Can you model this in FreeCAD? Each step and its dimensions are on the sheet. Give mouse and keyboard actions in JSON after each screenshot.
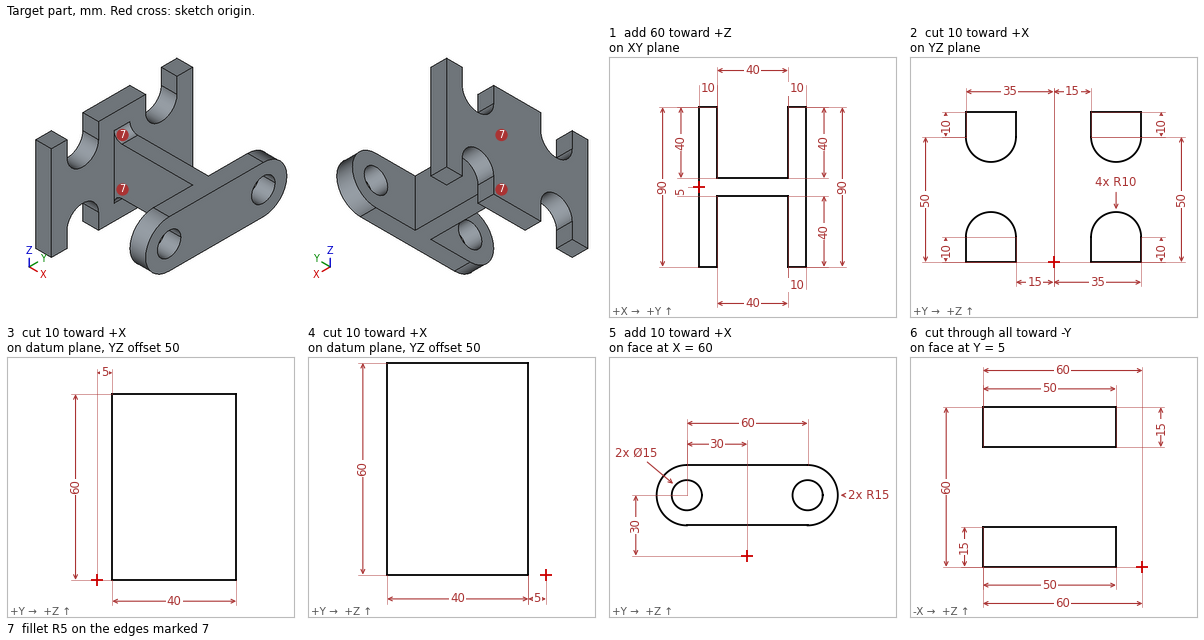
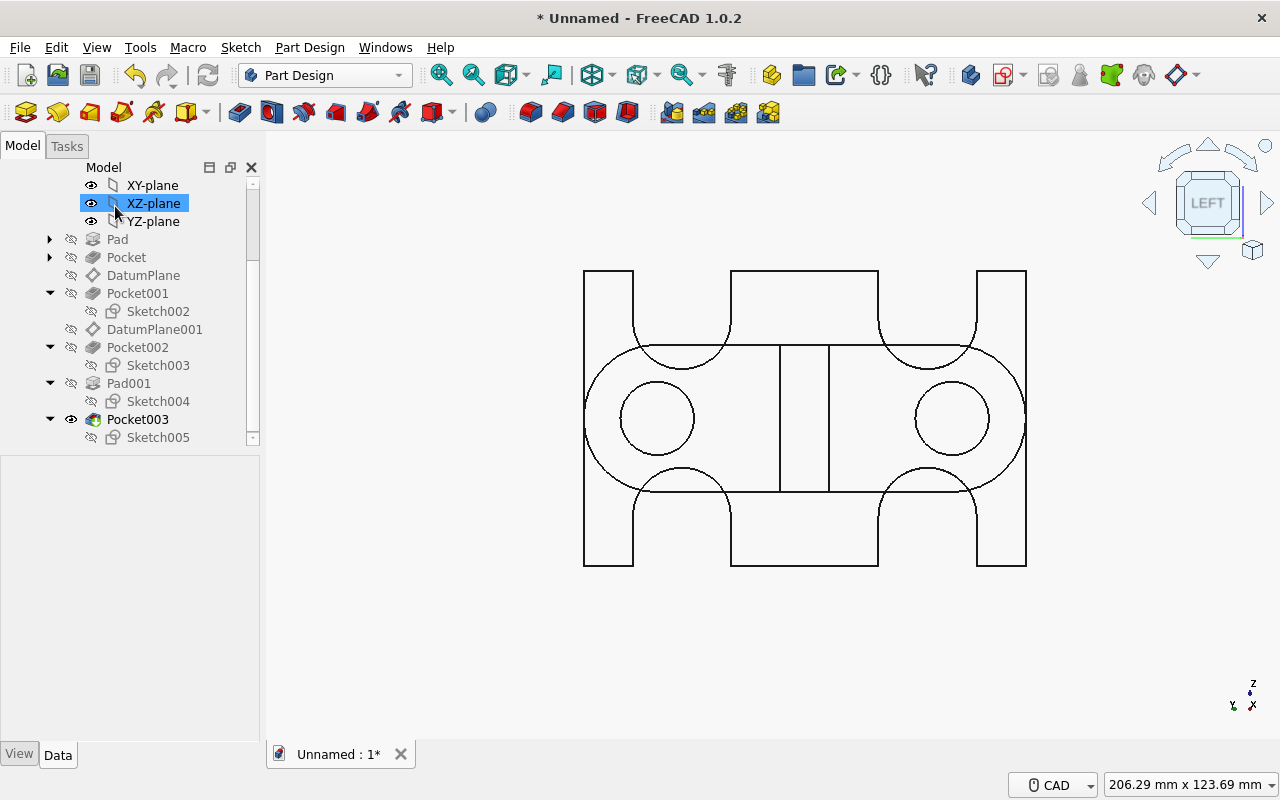
{"action": "key", "text": "0"}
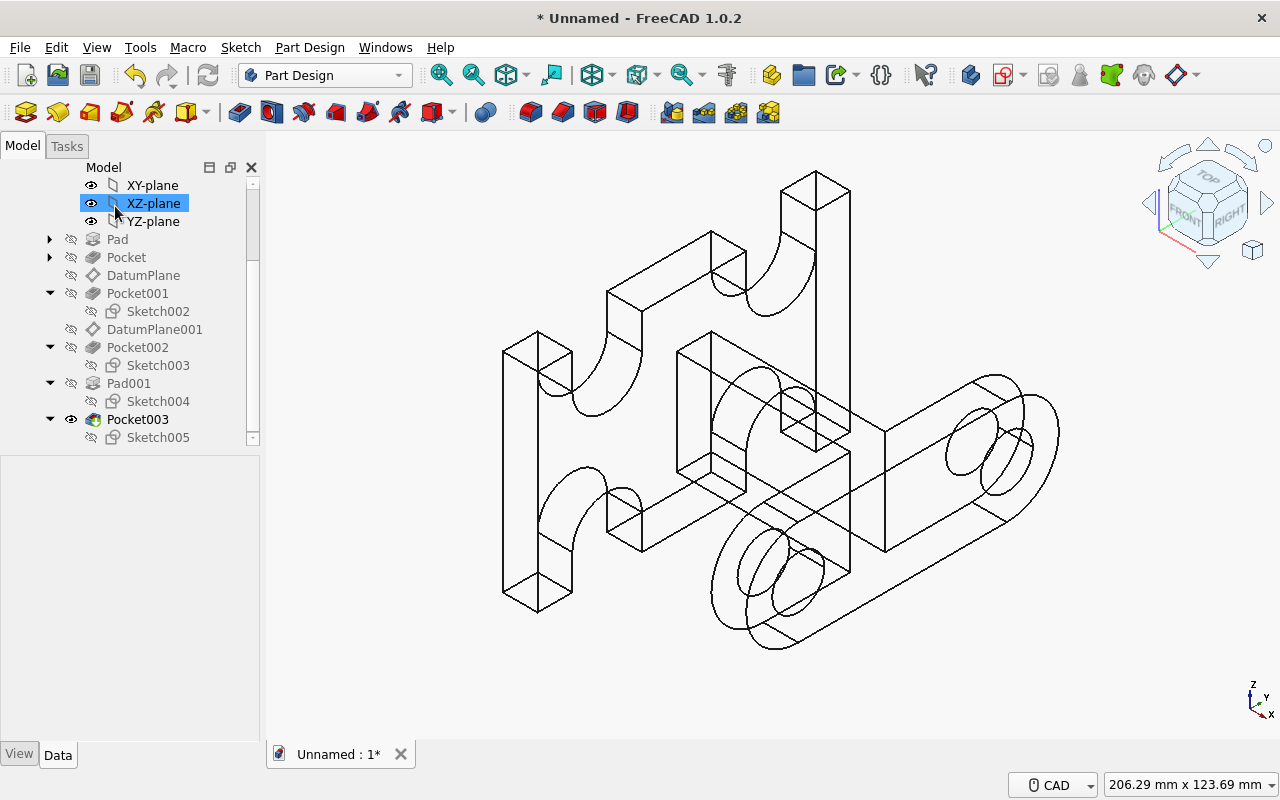
{"action": "left_click", "coordinate": [694, 461]}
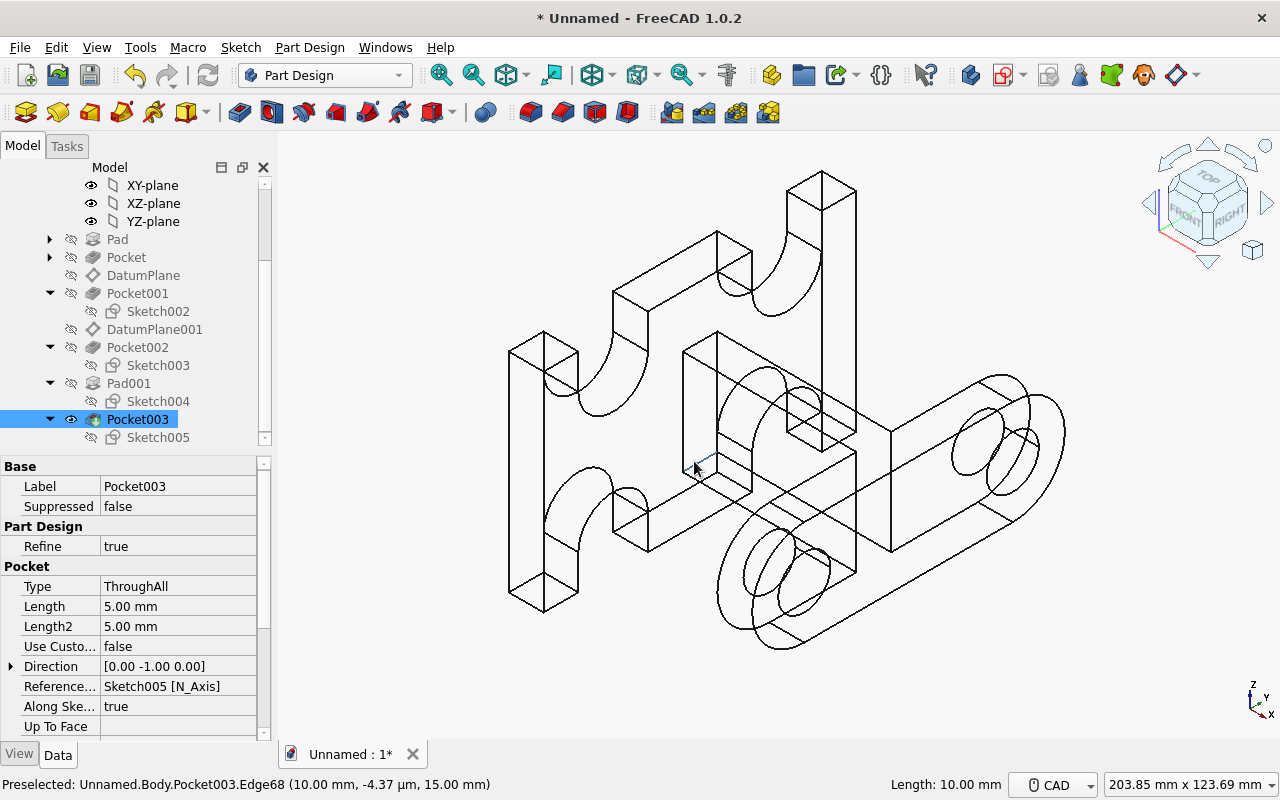
{"action": "left_click", "coordinate": [700, 341], "text": "ctrl"}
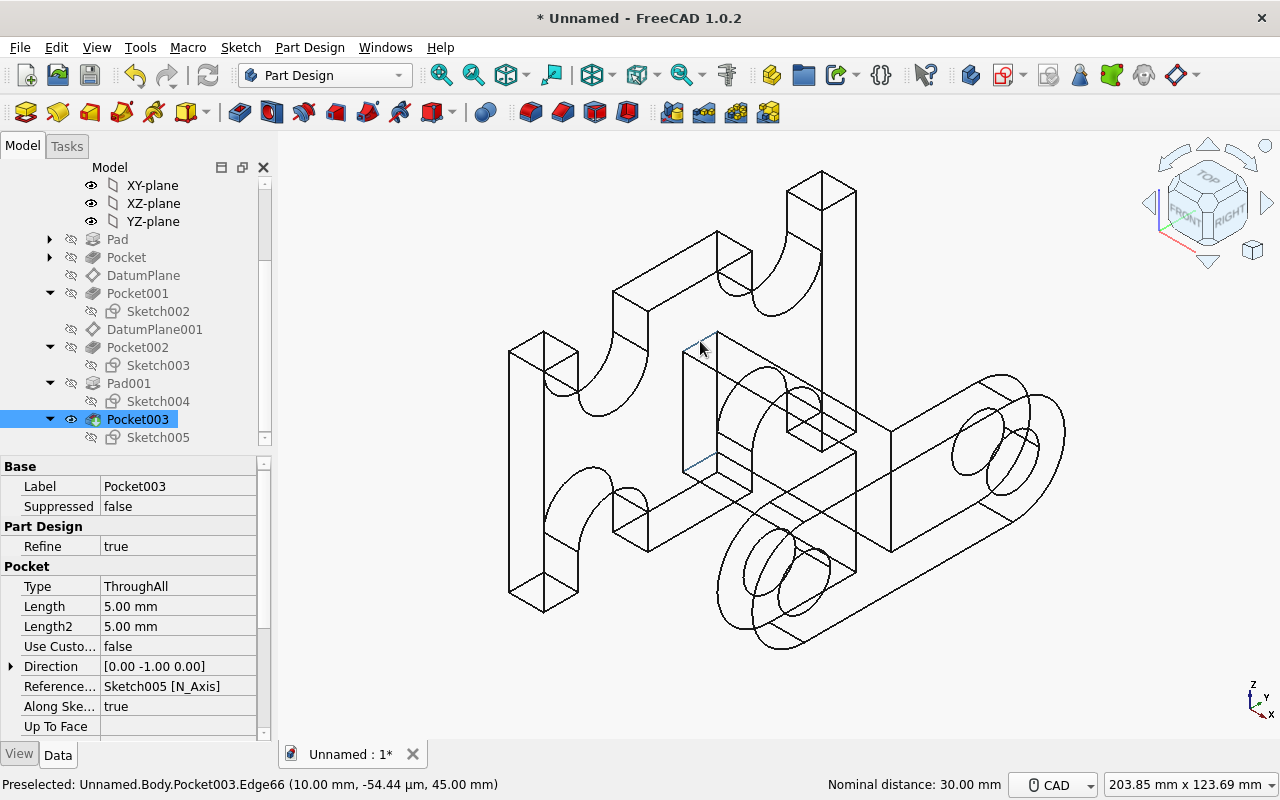
{"action": "key", "text": "v 1"}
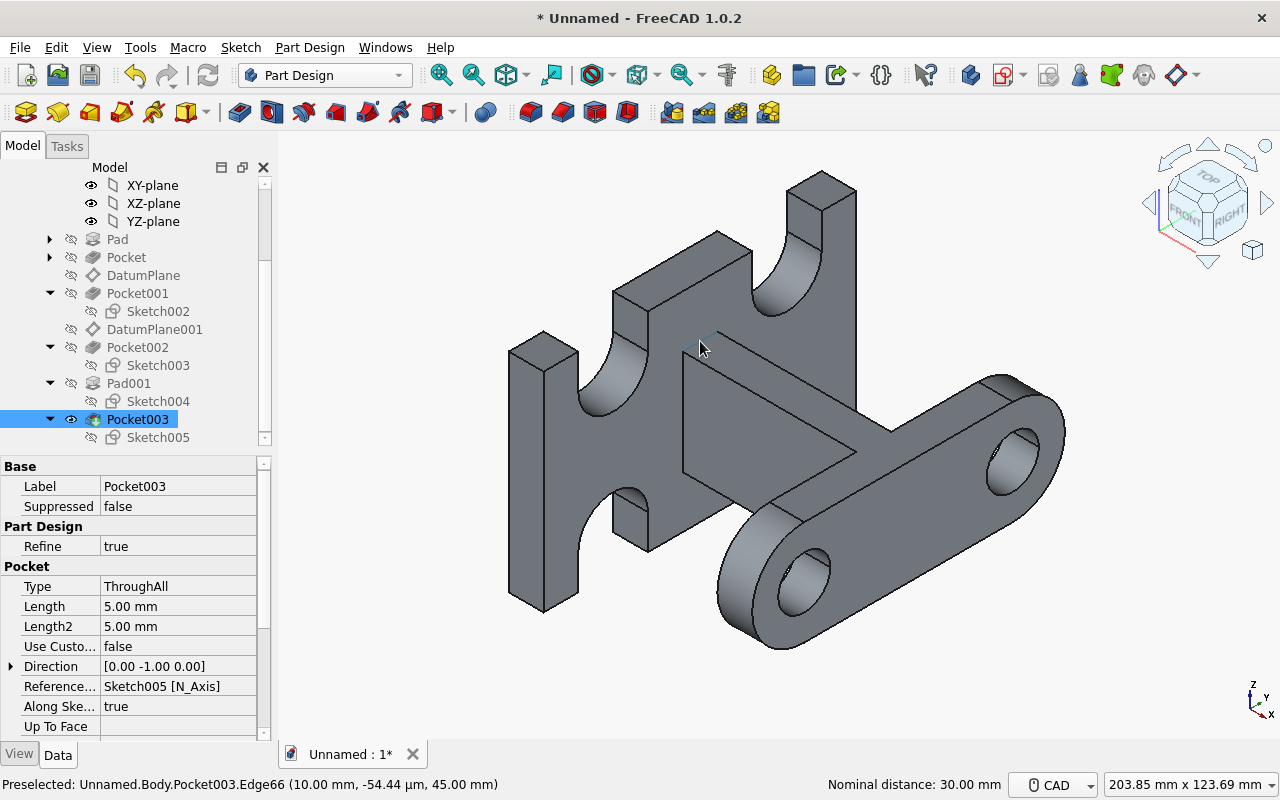
{"action": "left_click", "coordinate": [532, 112]}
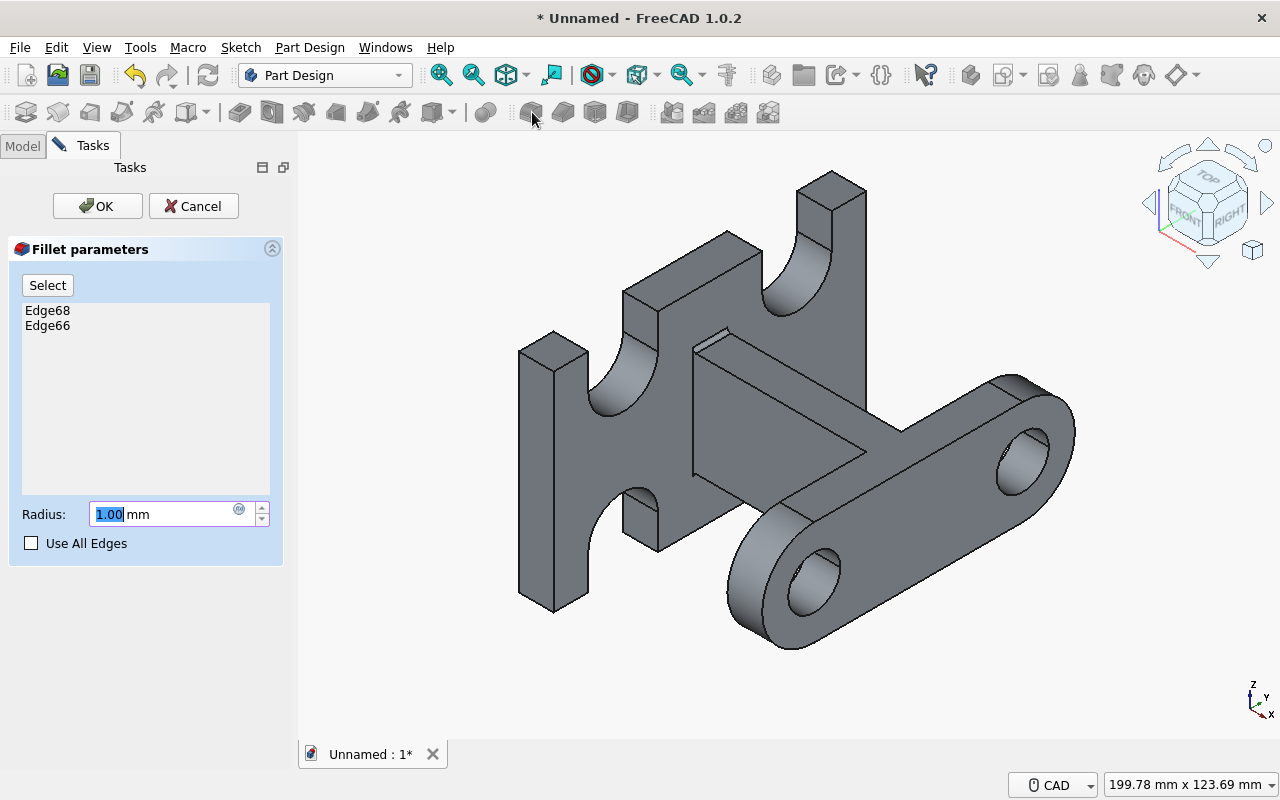
{"action": "type", "text": "5"}
{"action": "key", "text": "Tab"}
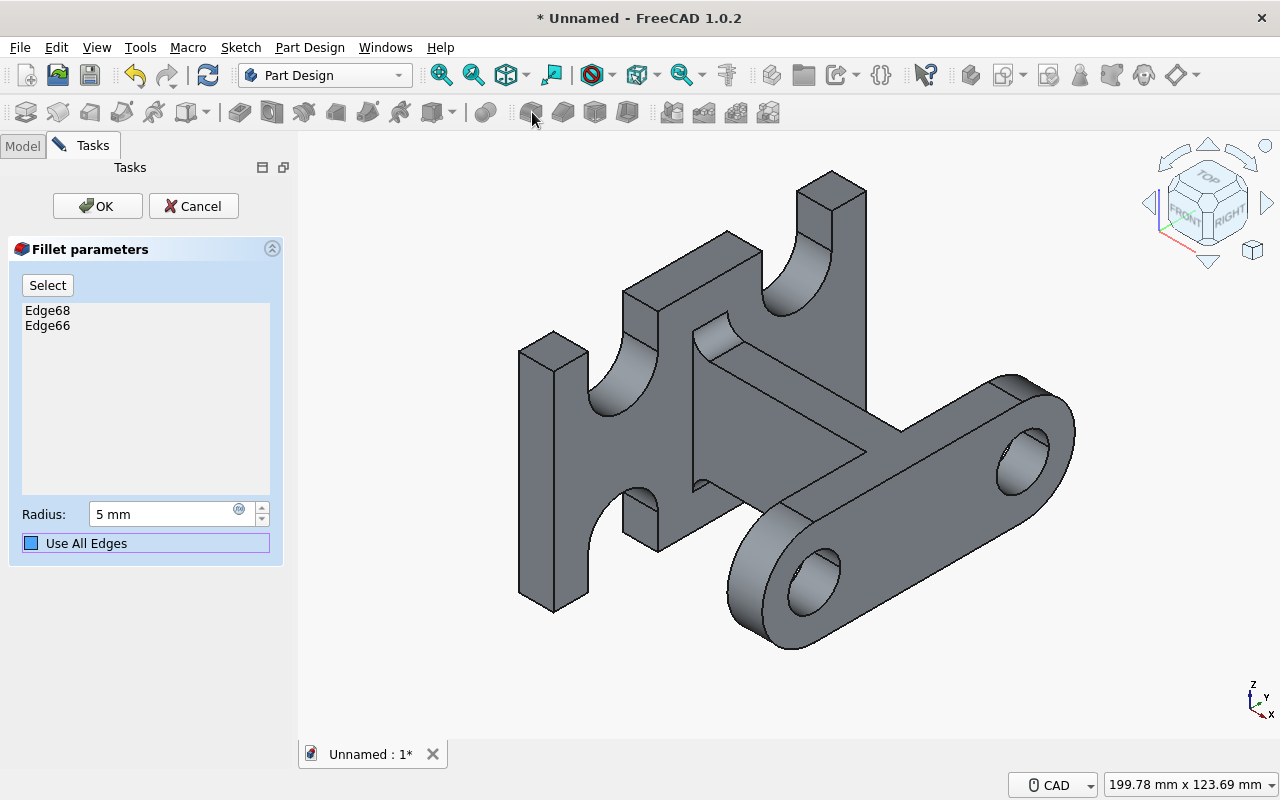
{"action": "left_click", "coordinate": [98, 206]}